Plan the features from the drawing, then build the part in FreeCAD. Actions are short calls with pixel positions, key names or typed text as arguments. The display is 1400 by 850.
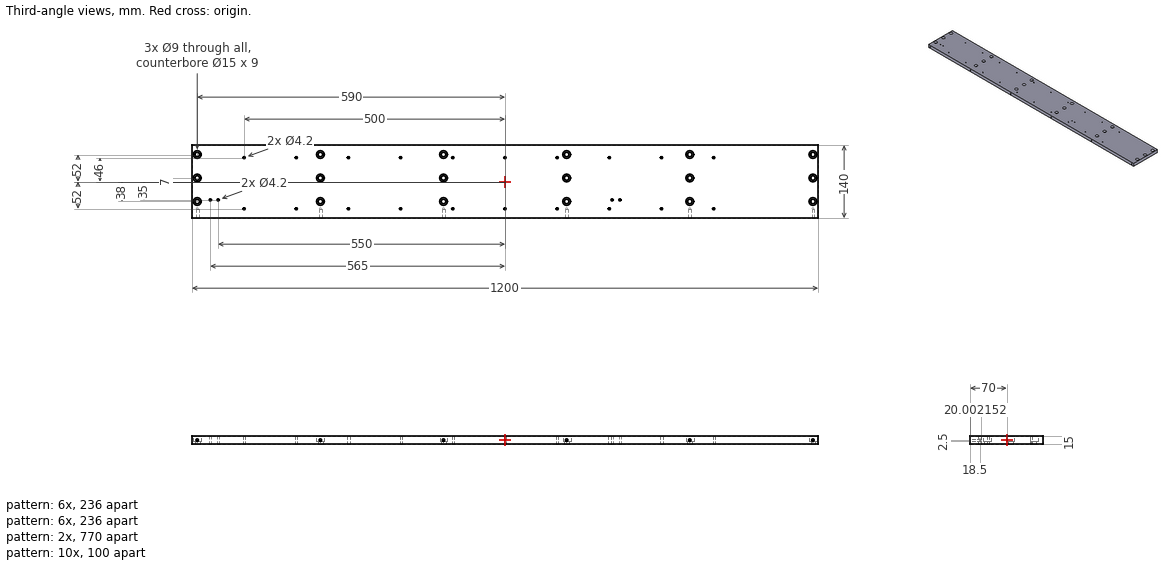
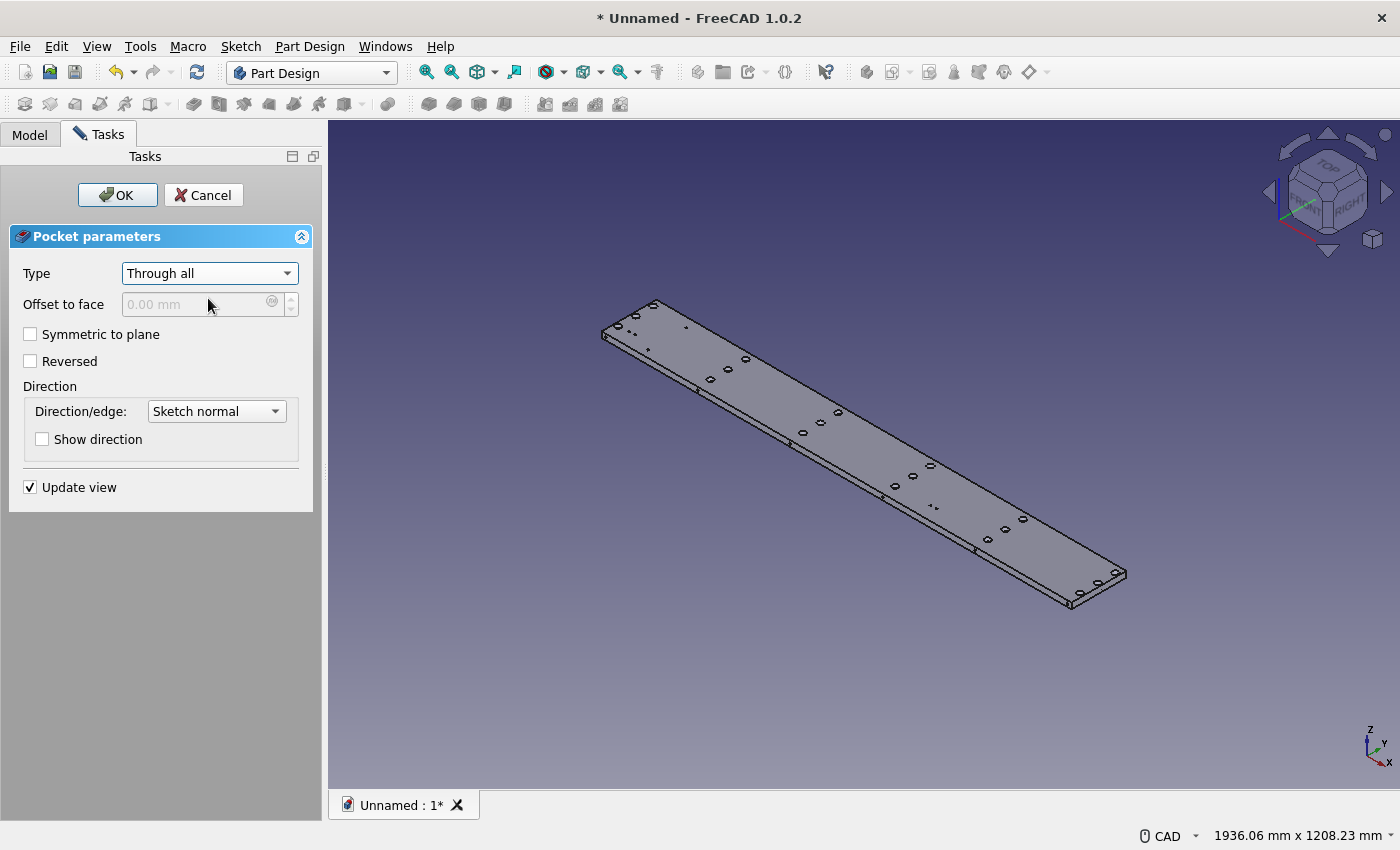
click(118, 195)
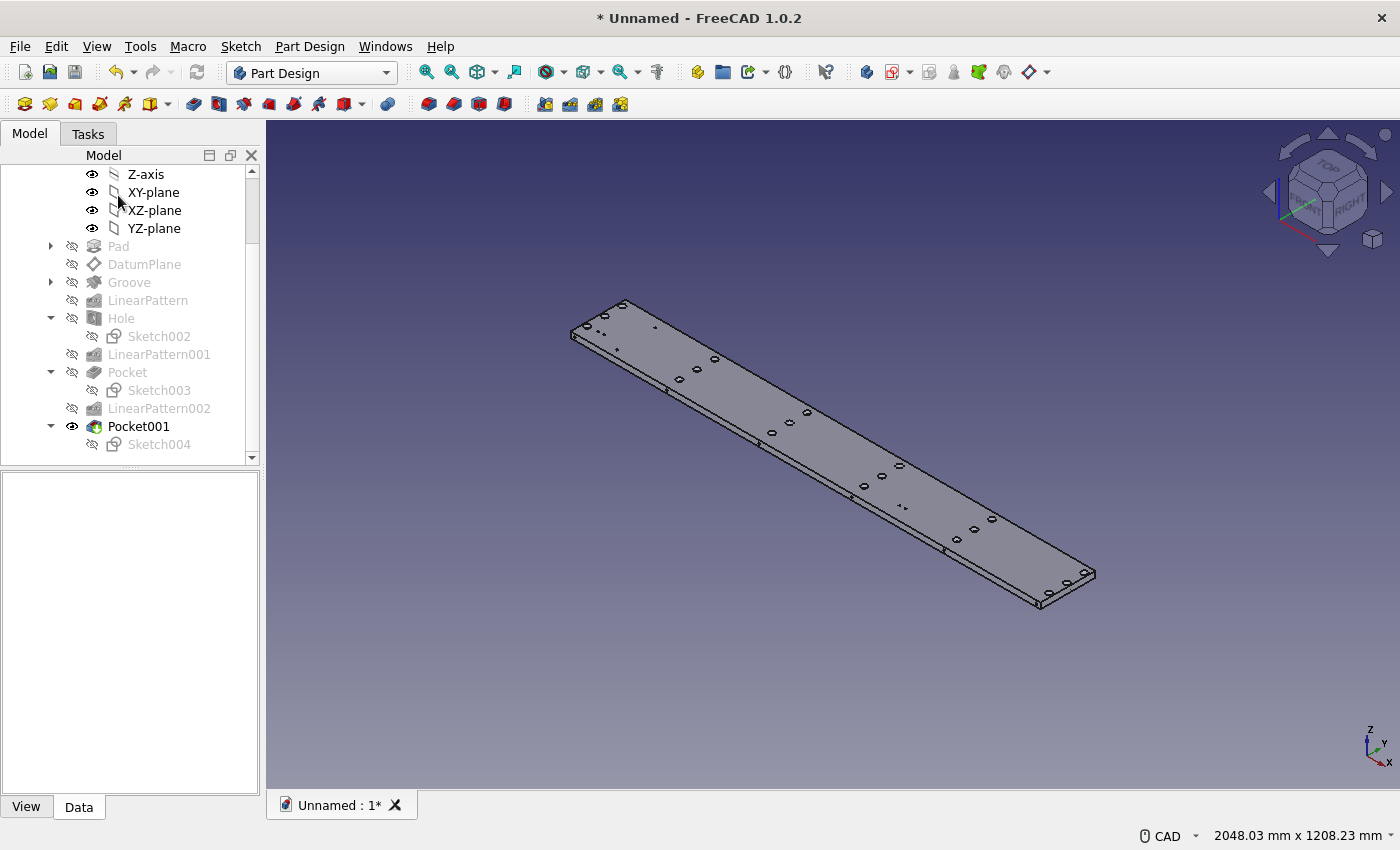
click(117, 426)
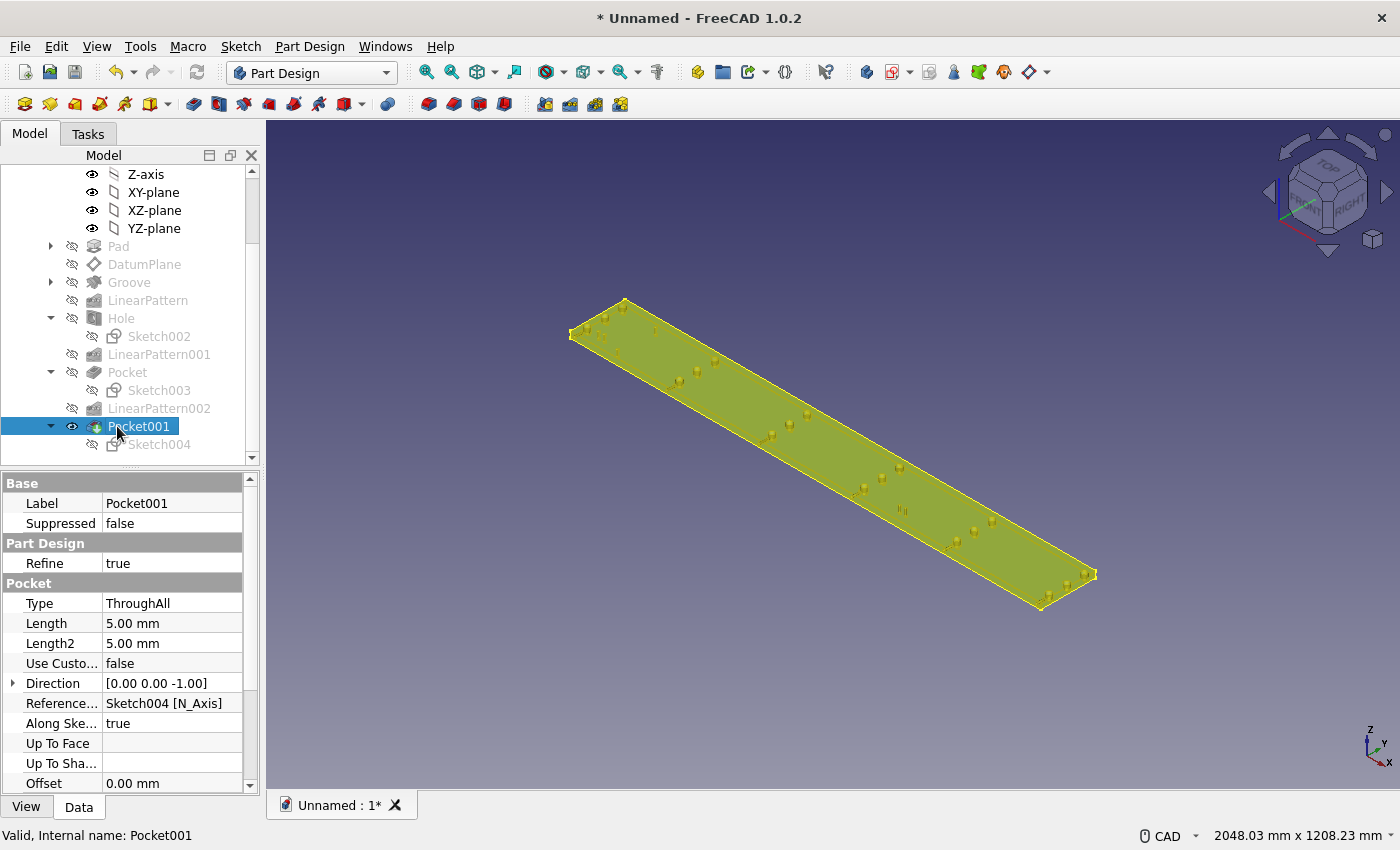
click(570, 104)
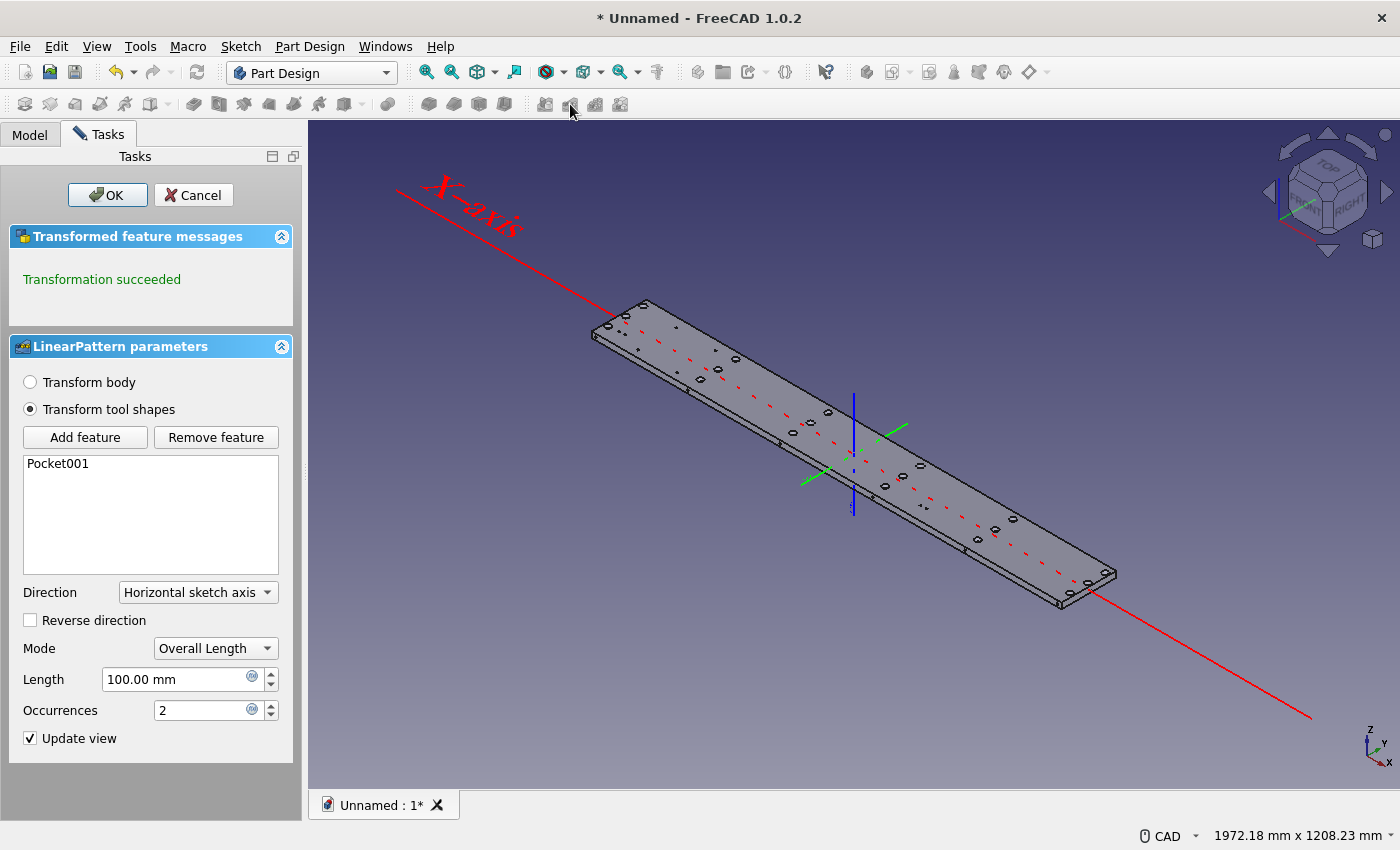
click(199, 592)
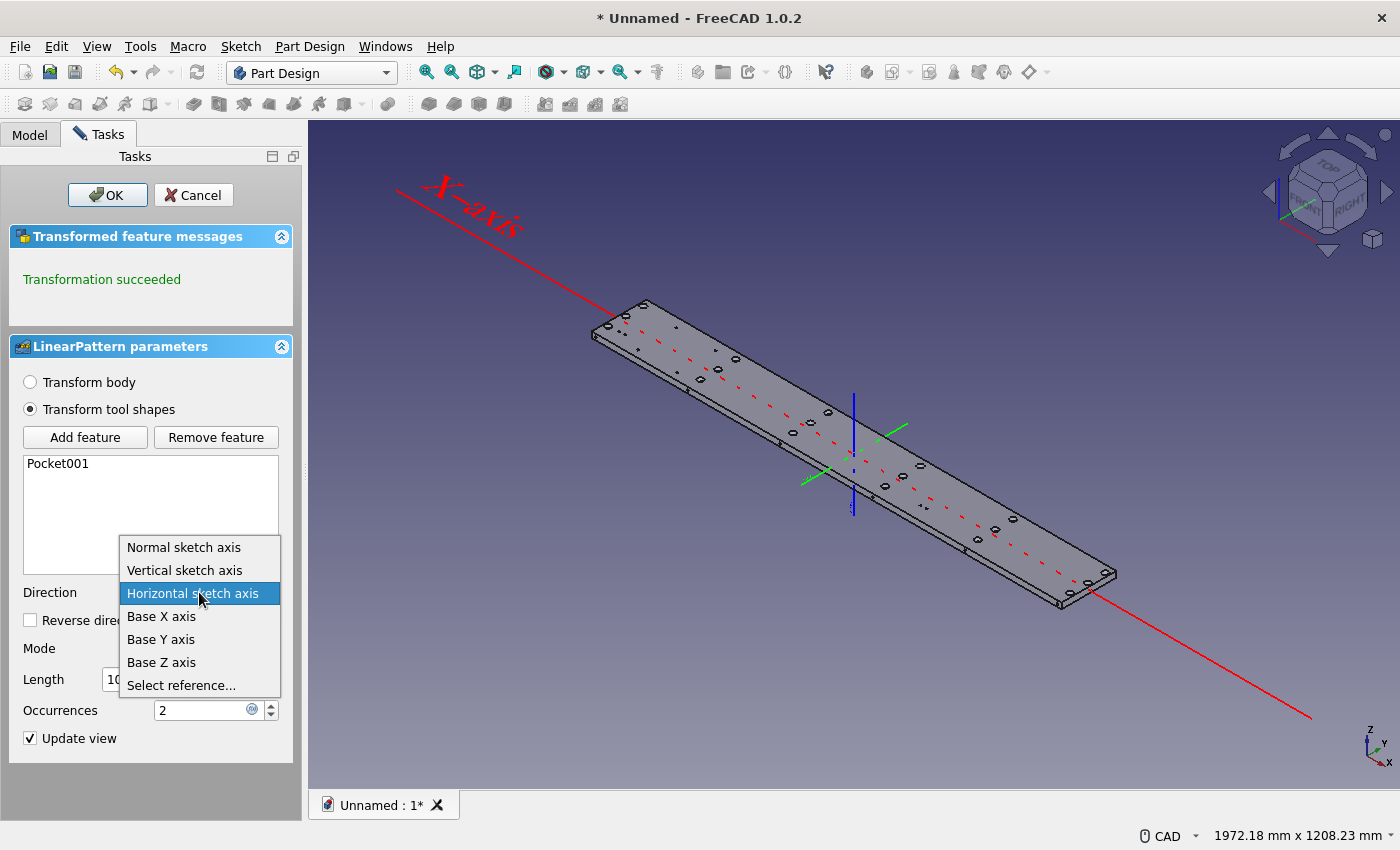
click(198, 616)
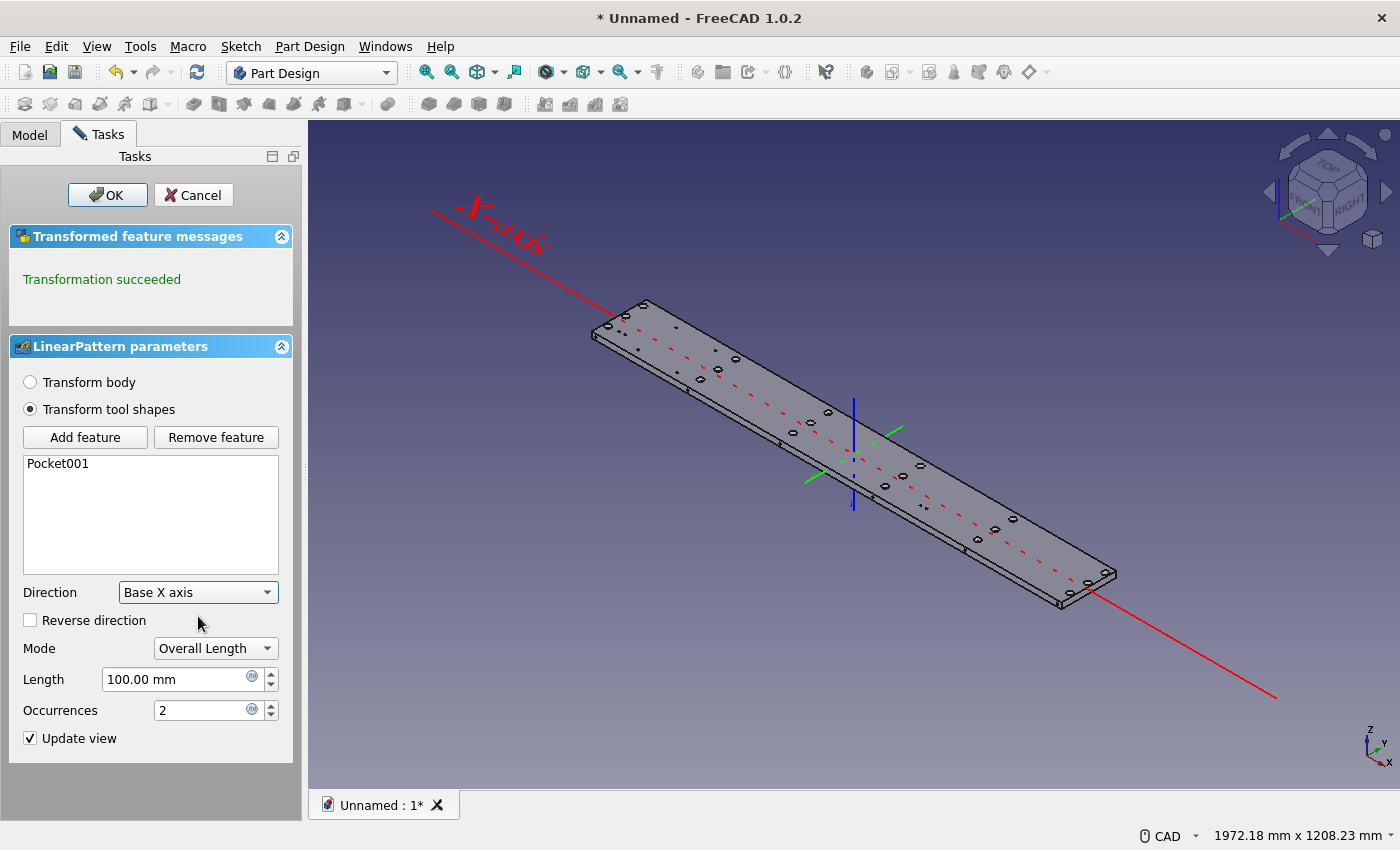
click(216, 648)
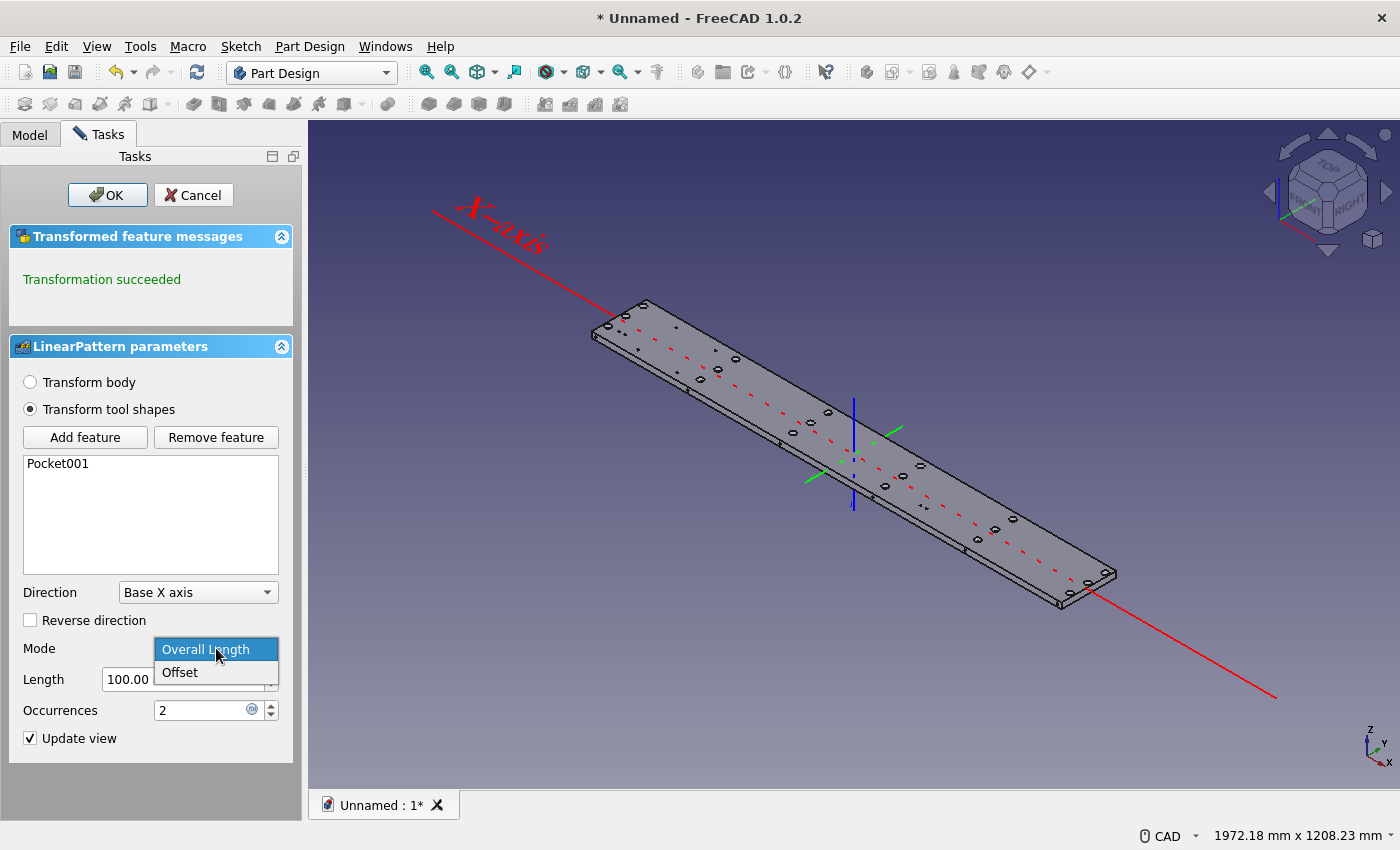
click(214, 672)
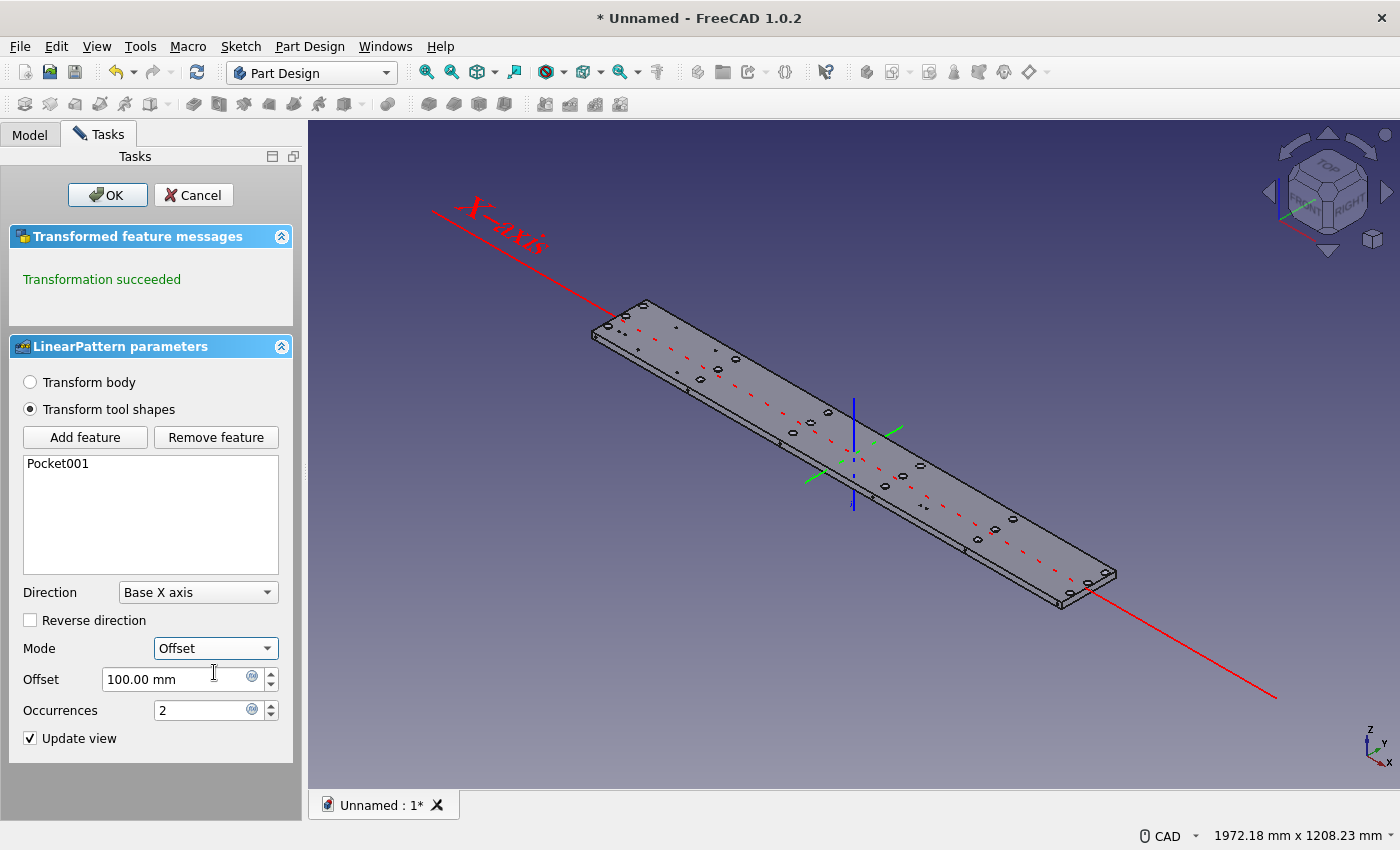
triple_click(184, 680)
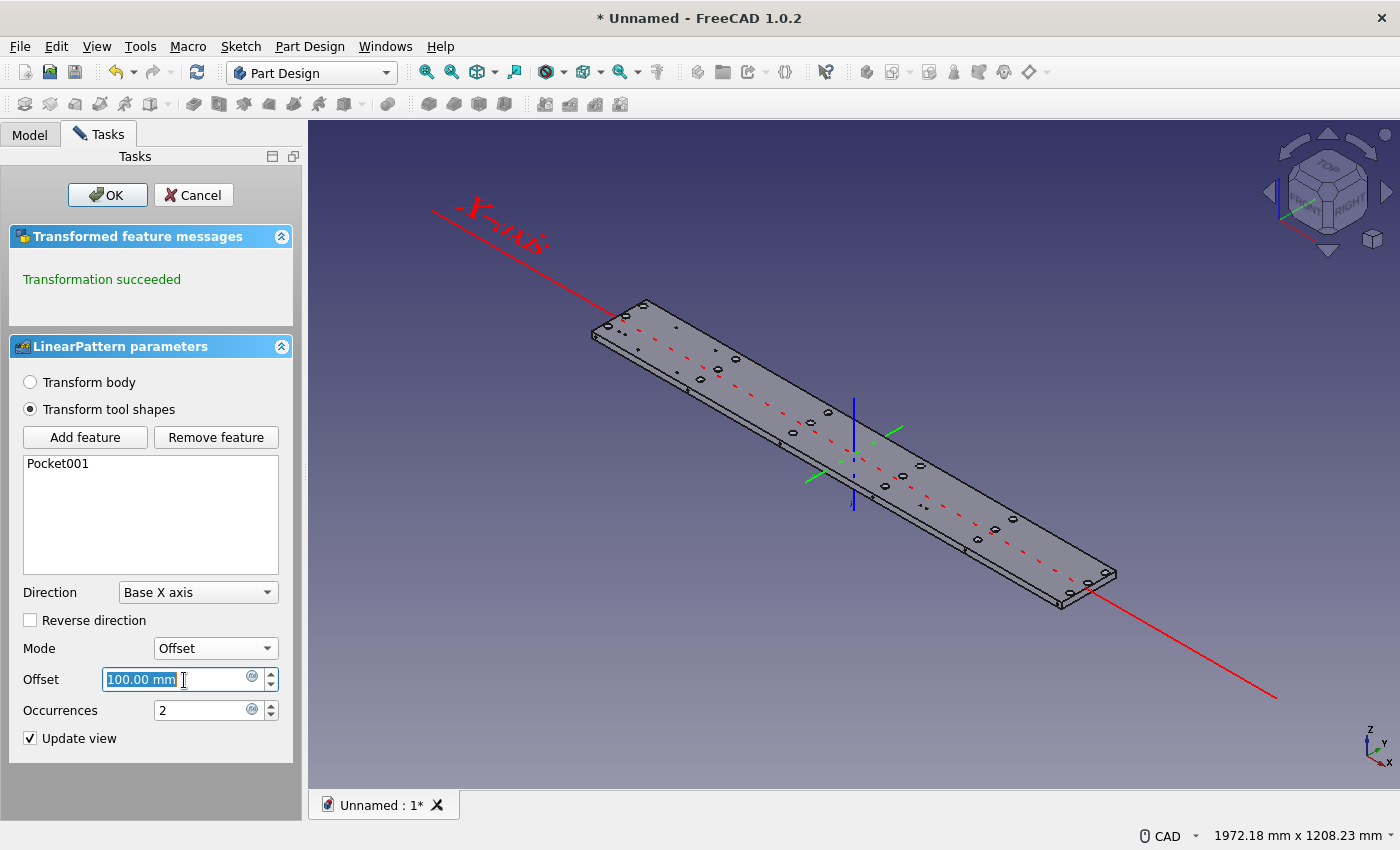
text(100)
key(Tab)